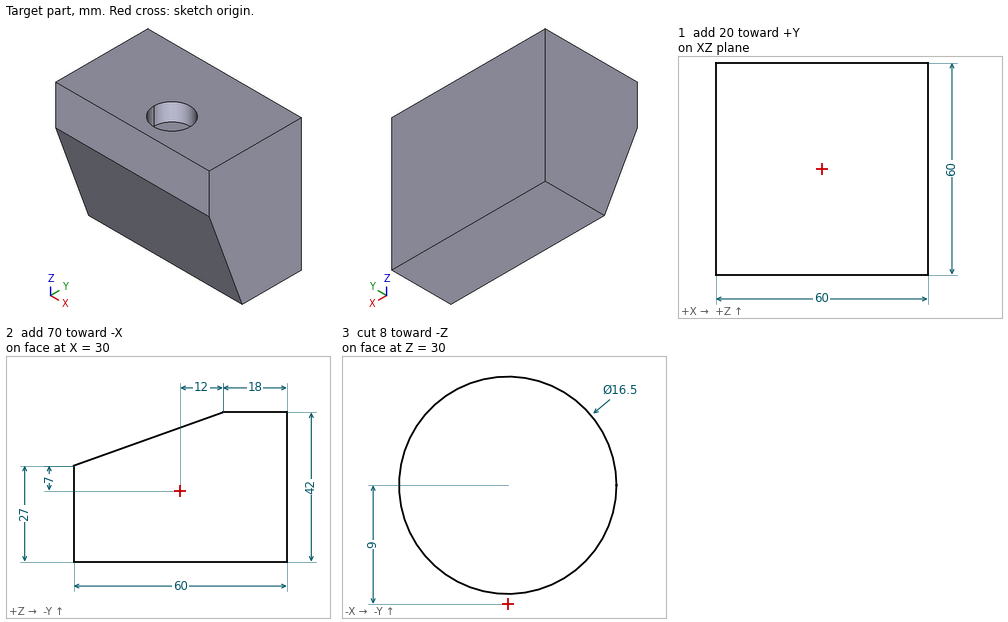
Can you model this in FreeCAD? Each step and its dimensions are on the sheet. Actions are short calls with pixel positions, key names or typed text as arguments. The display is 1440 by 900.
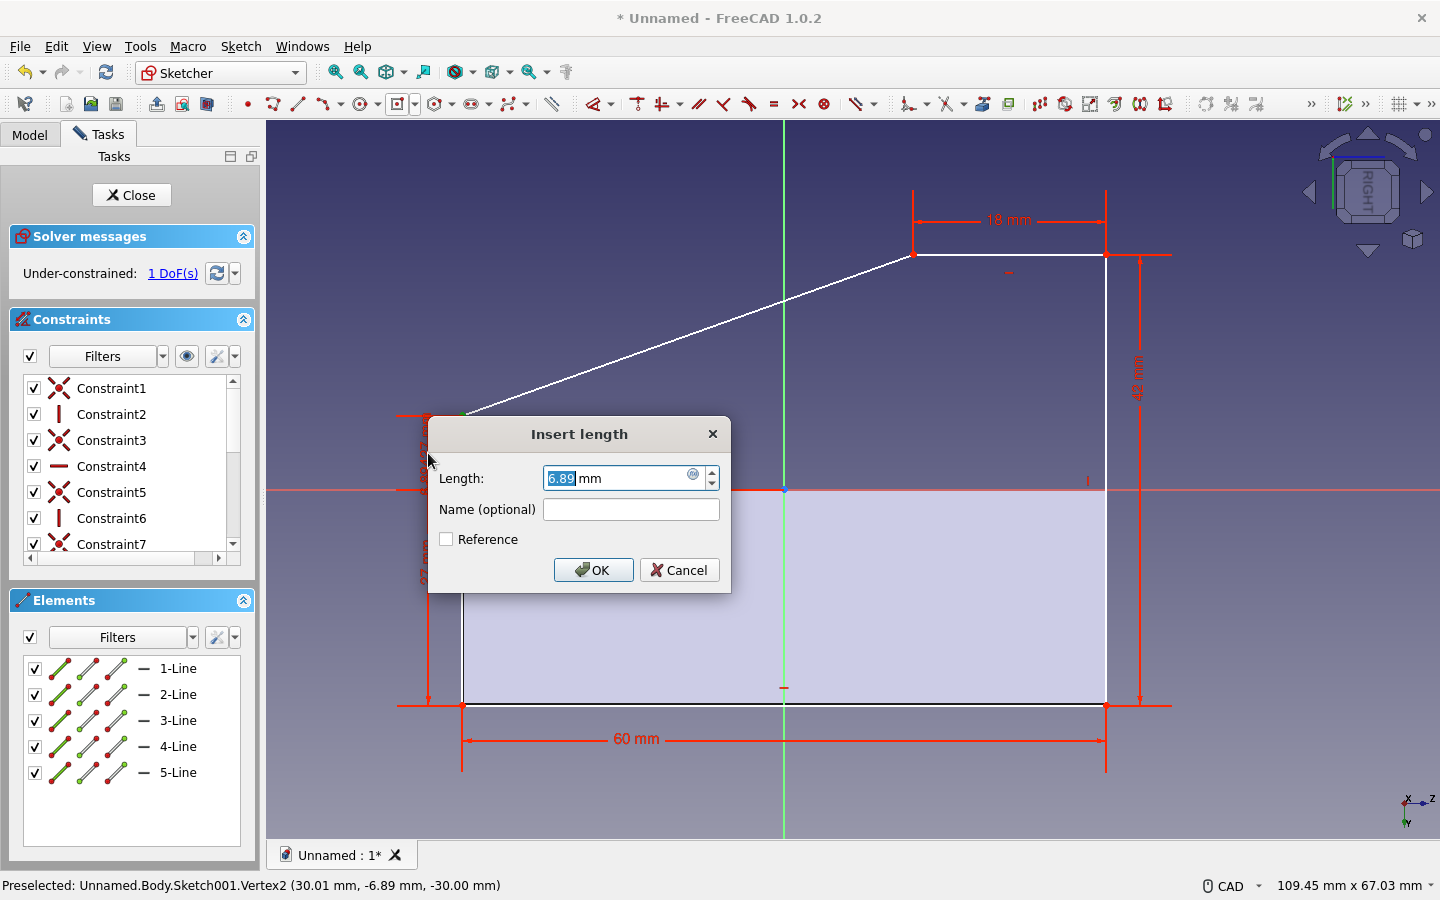
text(7)
key(Return)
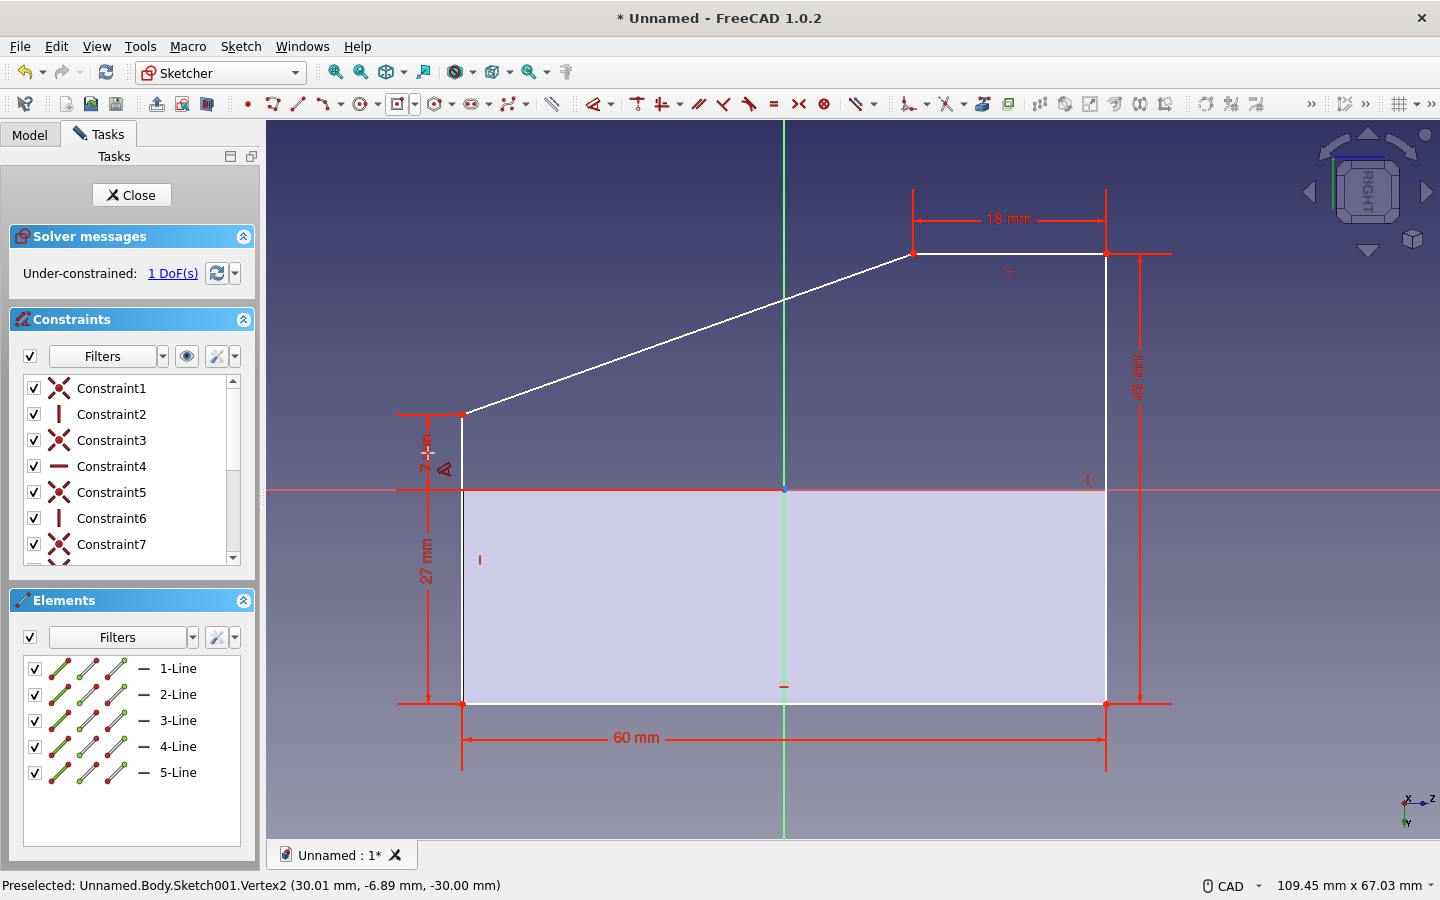
click(913, 254)
click(849, 220)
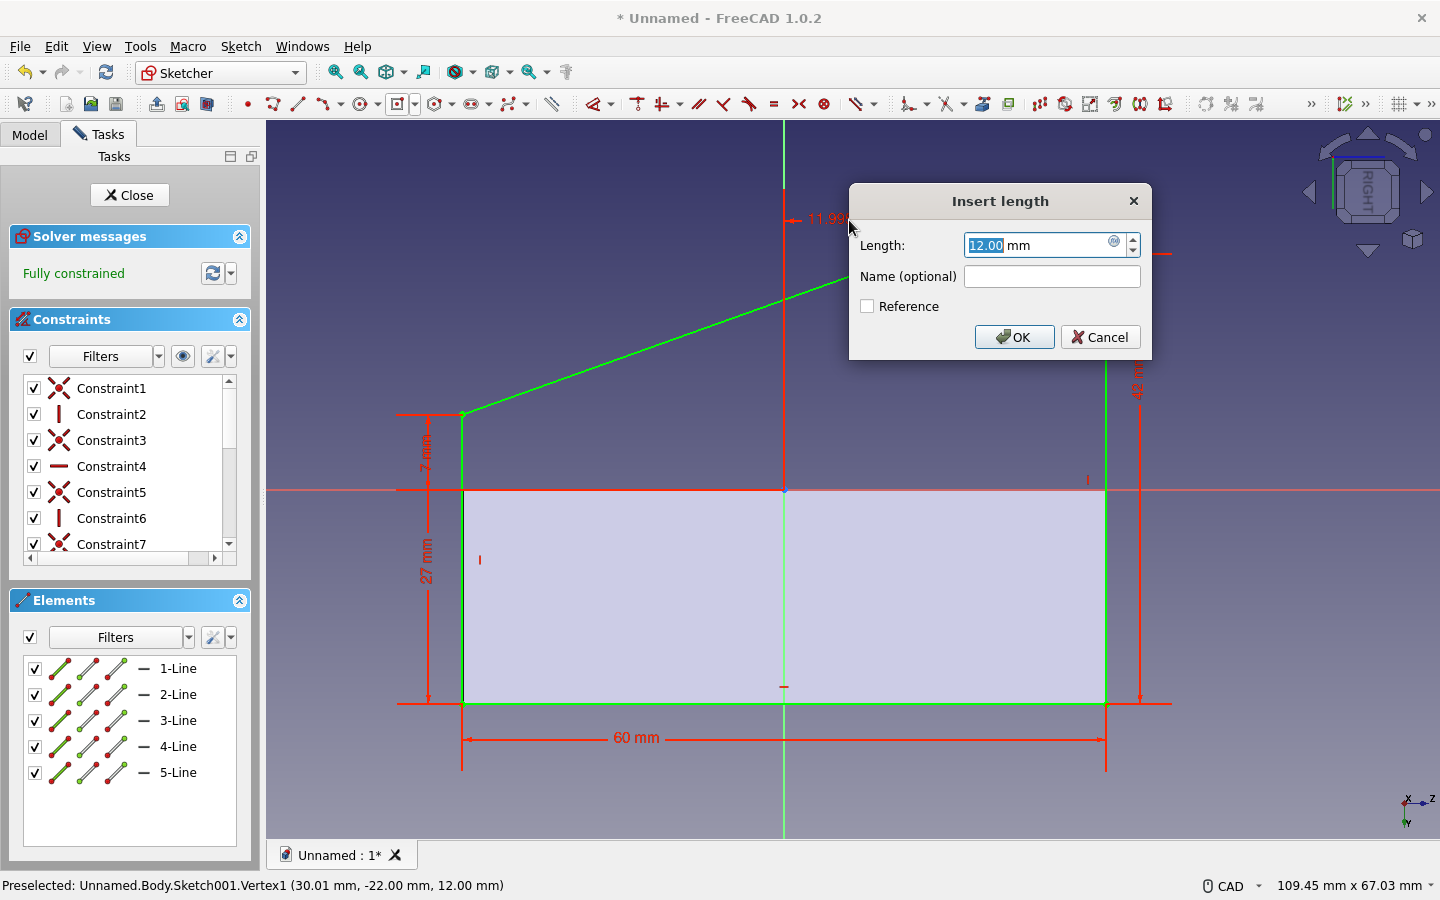
text(12)
key(Return)
key(Escape)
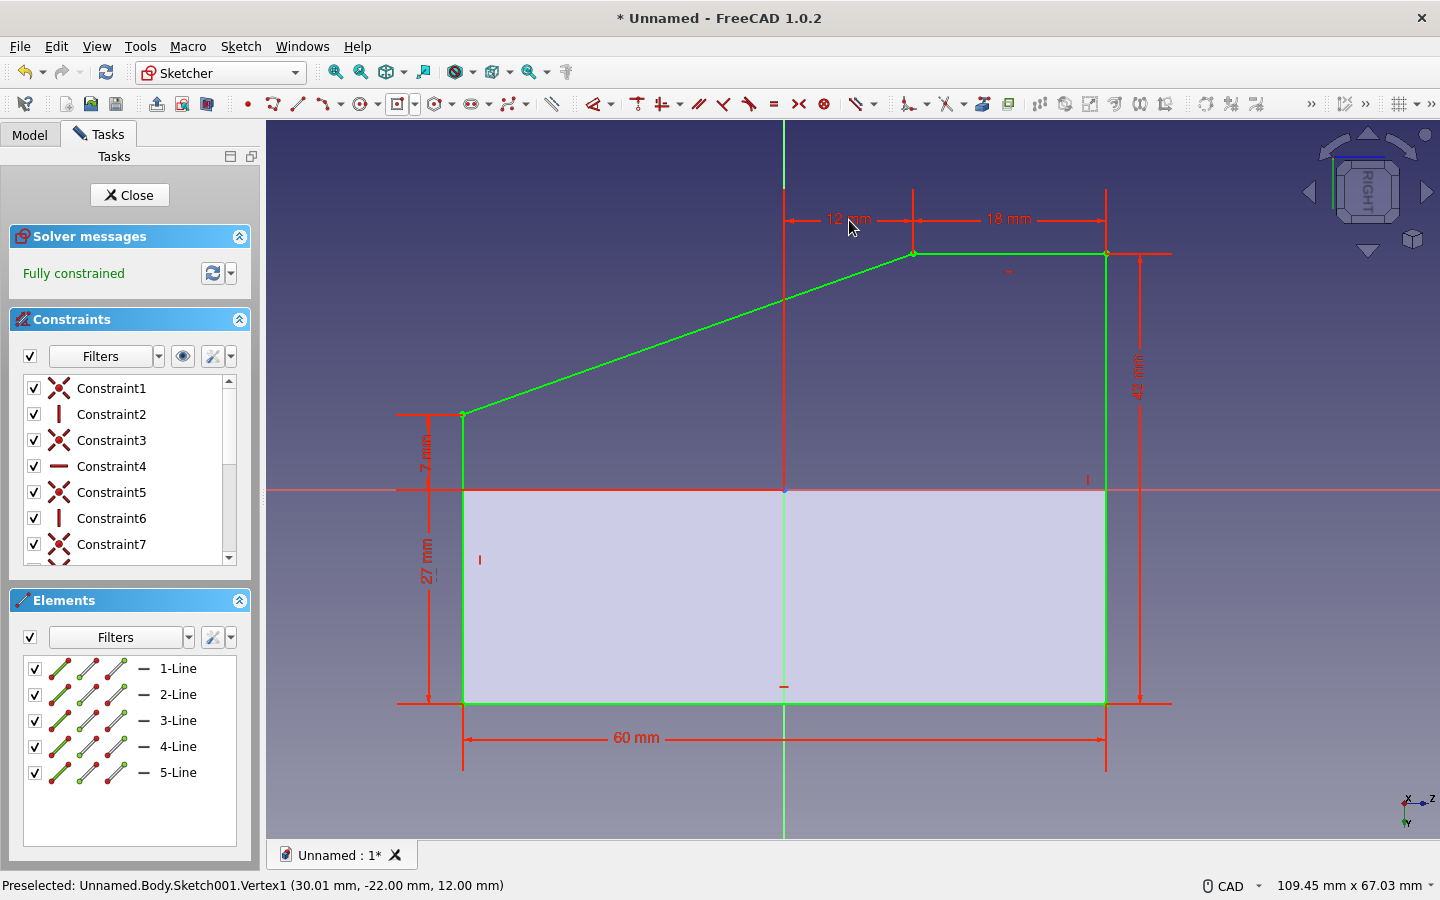
click(130, 195)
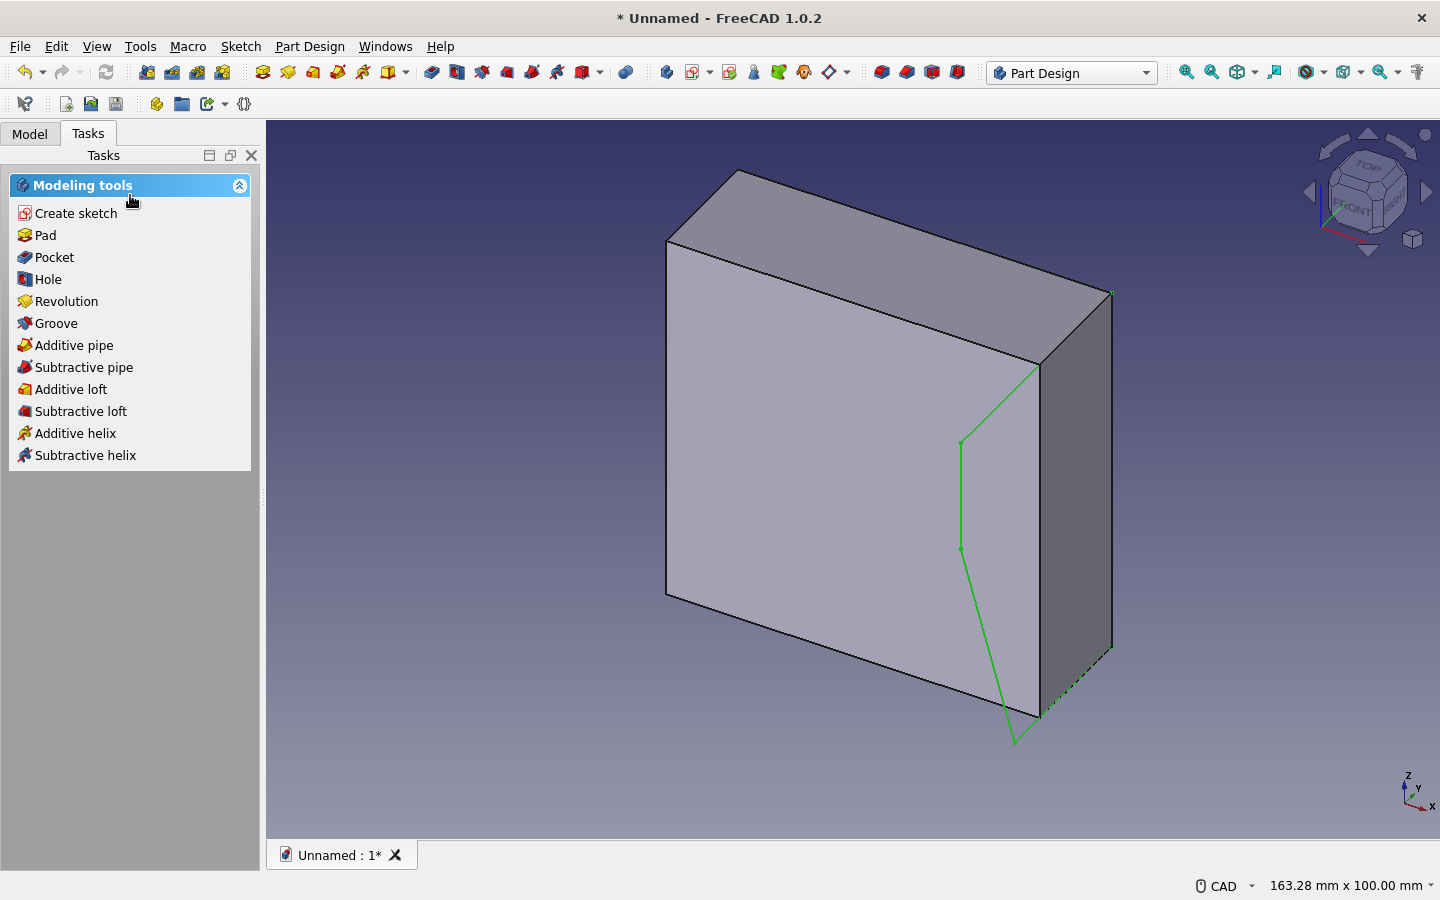
click(263, 72)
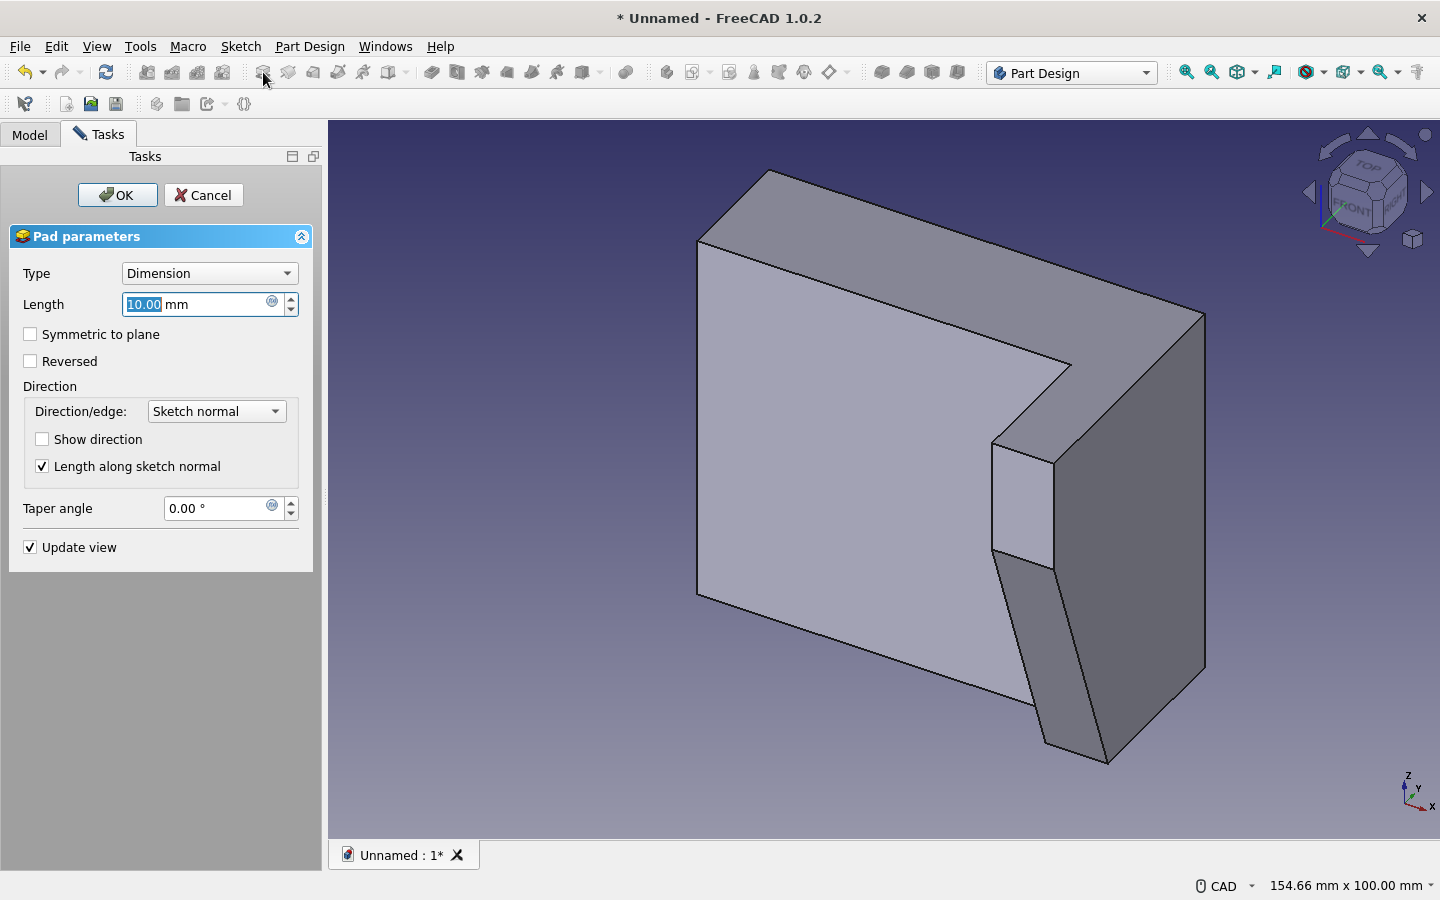
text(70)
key(Tab)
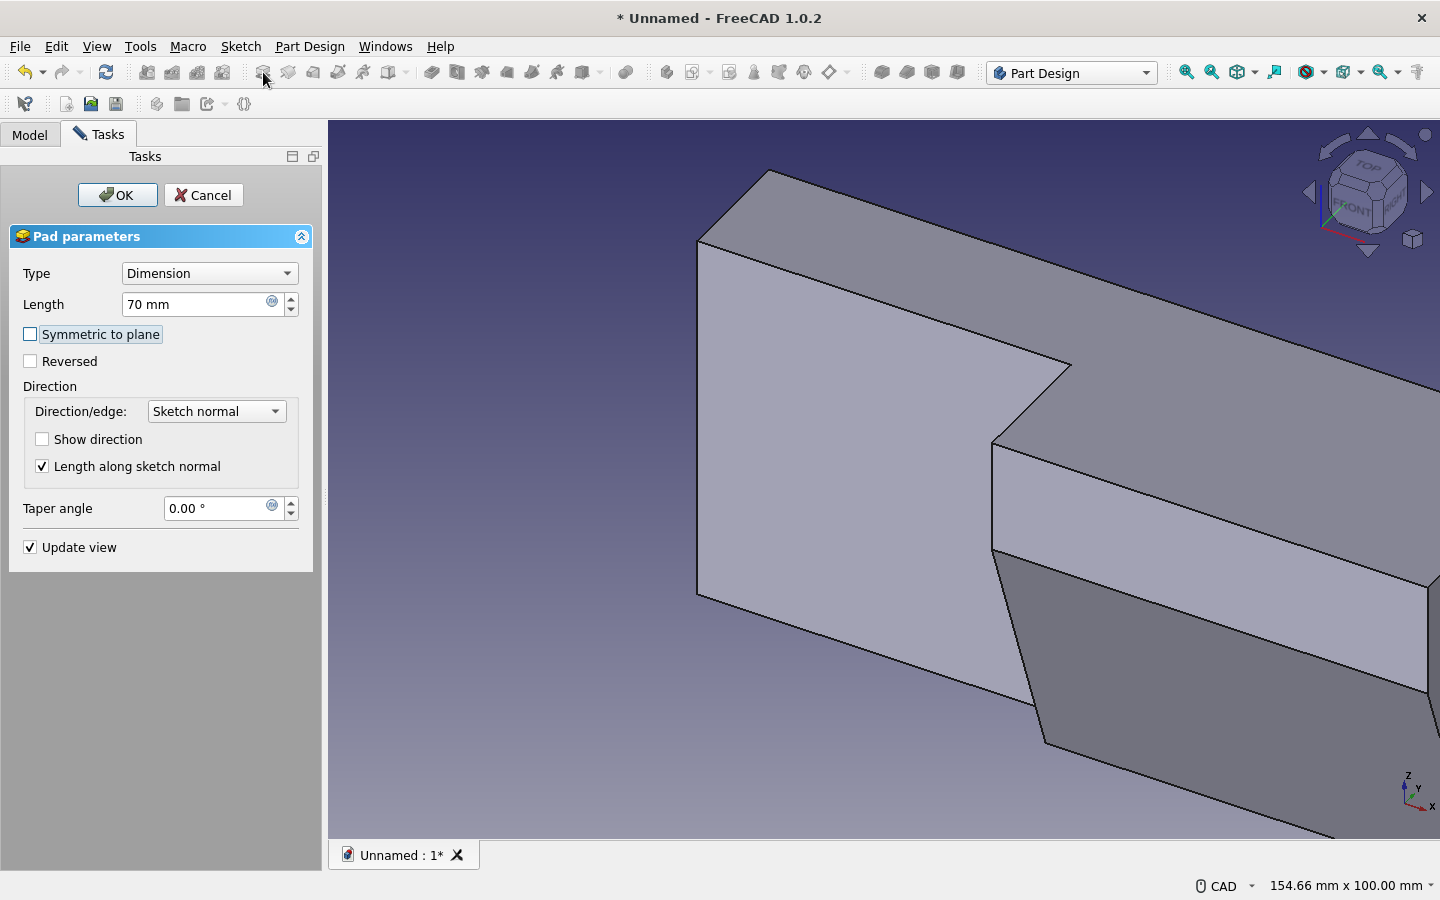
click(31, 361)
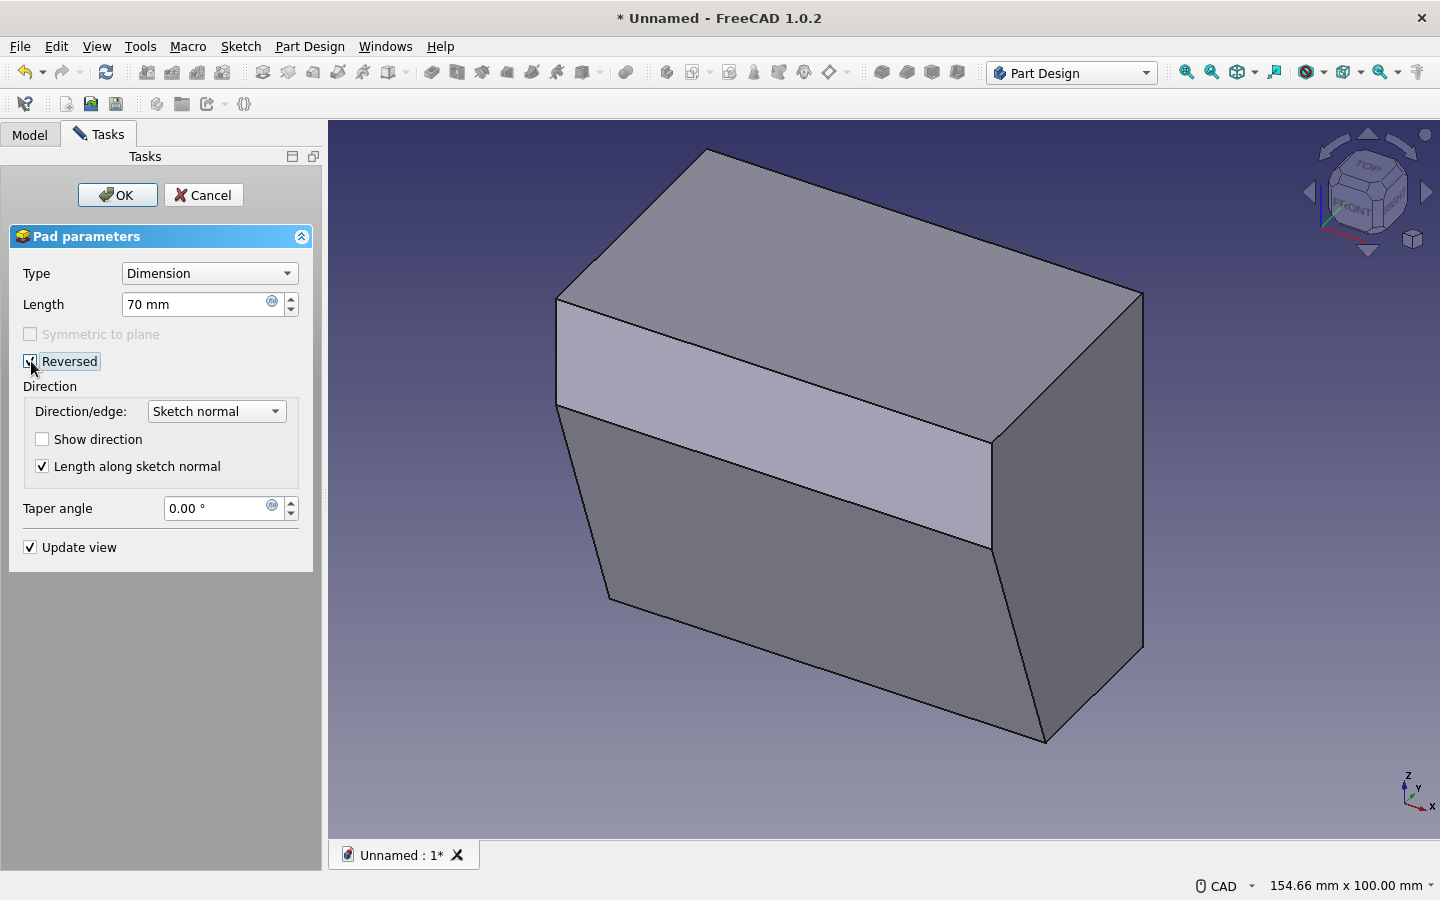
click(118, 195)